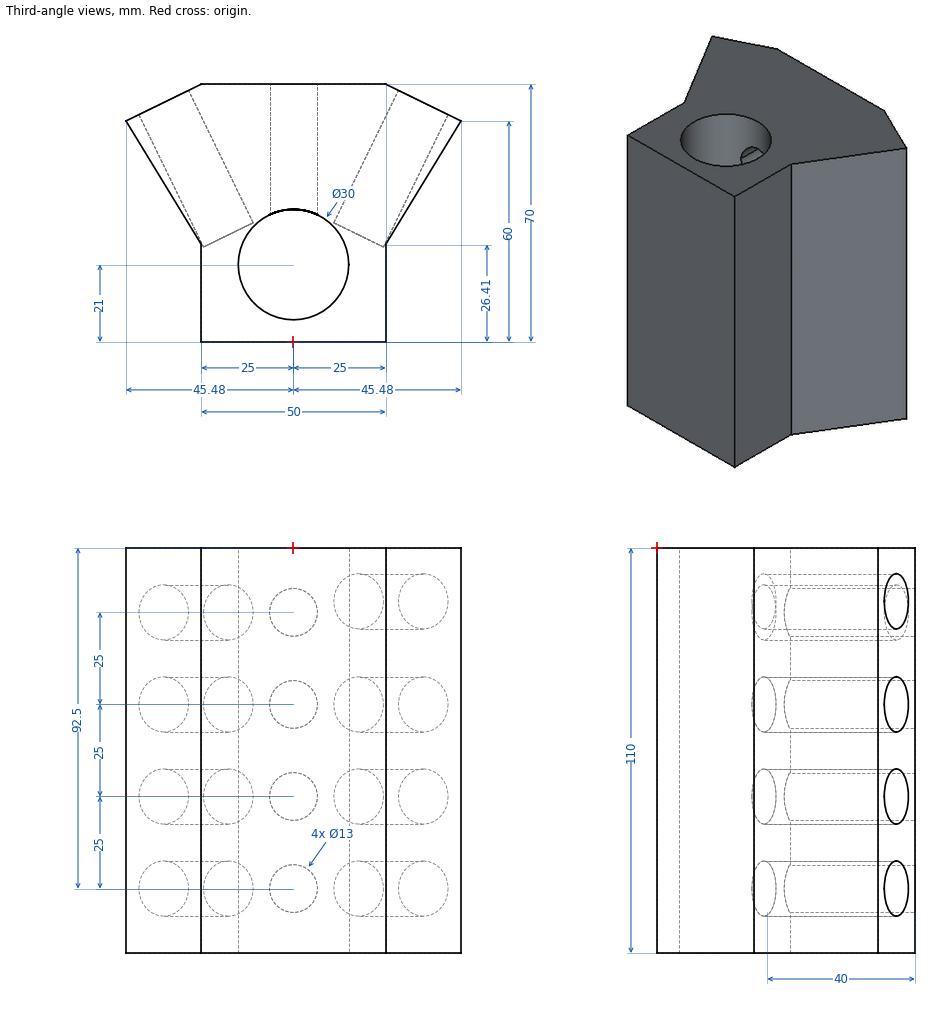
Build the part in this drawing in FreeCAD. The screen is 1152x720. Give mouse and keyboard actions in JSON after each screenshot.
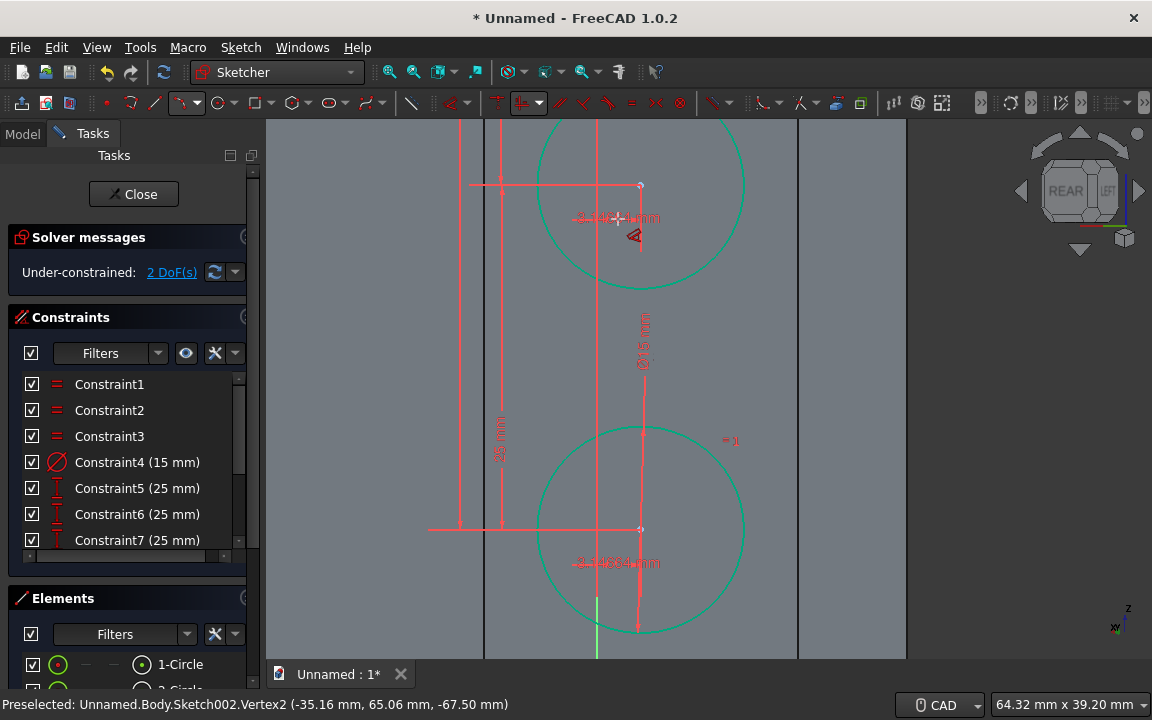
{"action": "scroll", "coordinate": [640, 535], "scroll_direction": "down", "scroll_amount": 7}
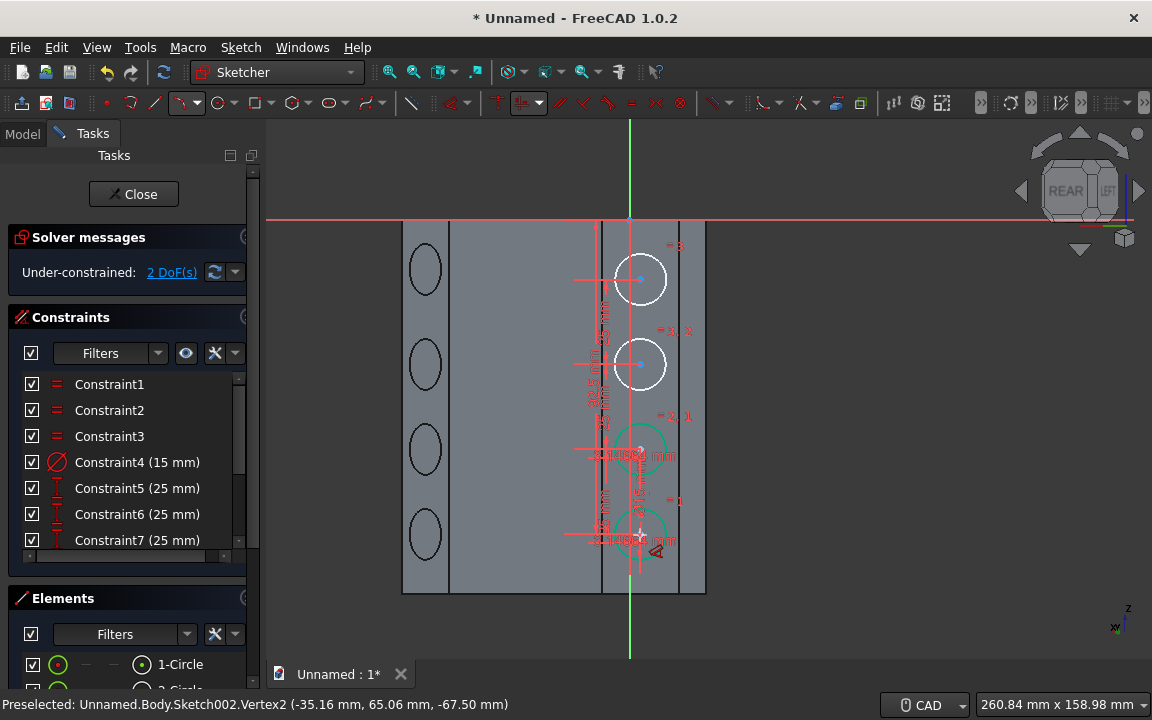
{"action": "scroll", "coordinate": [640, 364], "scroll_direction": "up", "scroll_amount": 7}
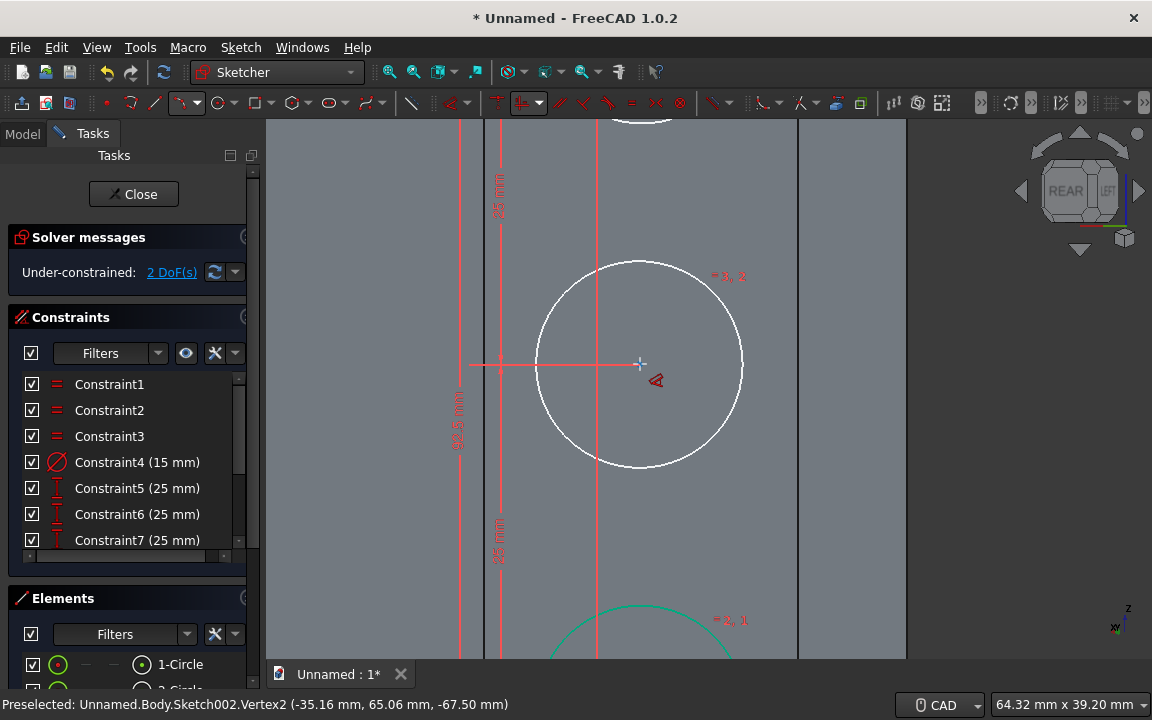
{"action": "left_click", "coordinate": [639, 365]}
{"action": "left_click", "coordinate": [618, 399]}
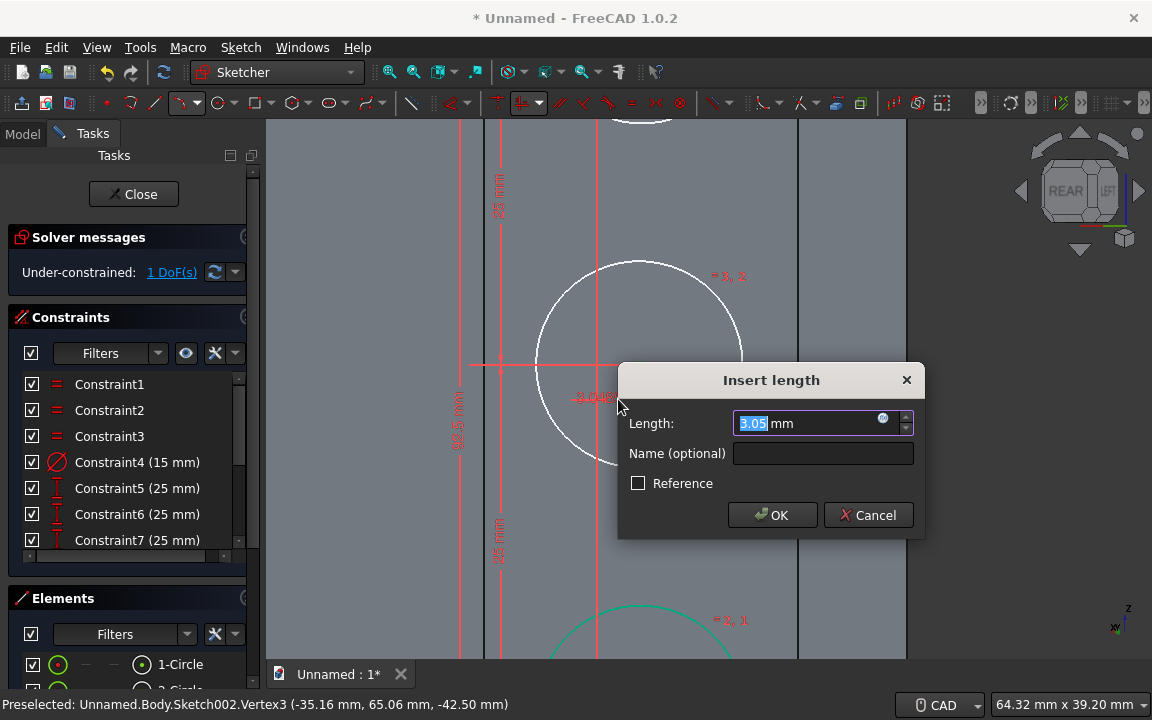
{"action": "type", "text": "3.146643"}
{"action": "key", "text": "Return"}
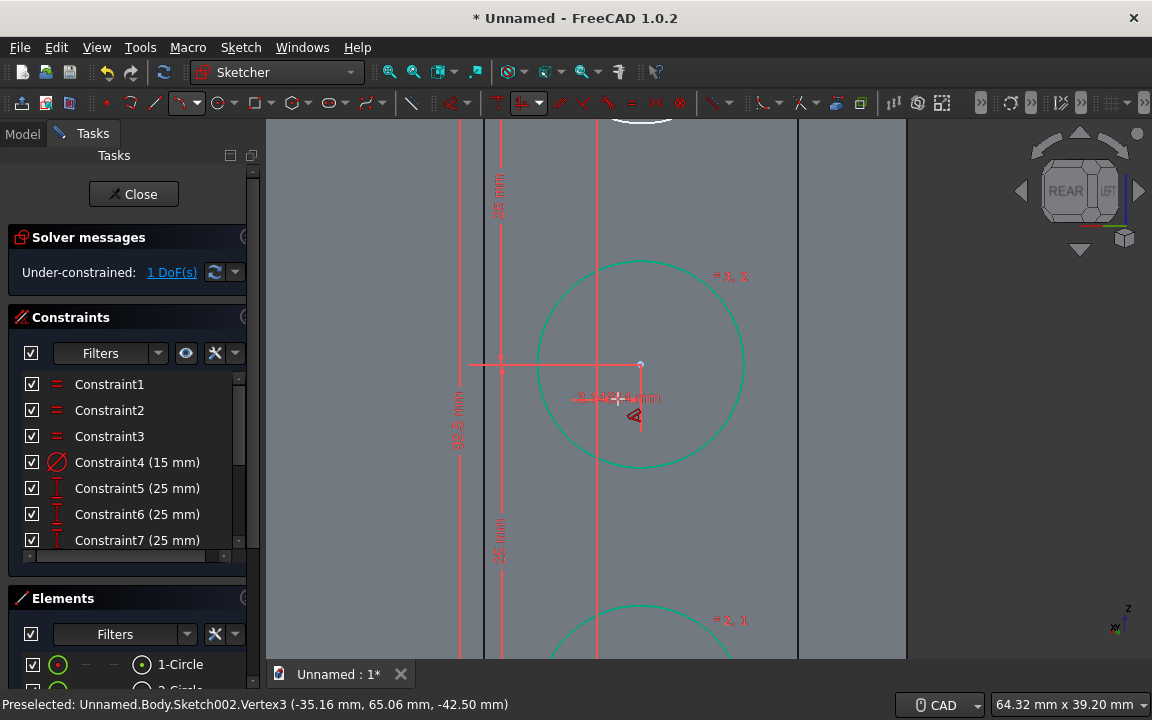
{"action": "scroll", "coordinate": [640, 363], "scroll_direction": "down", "scroll_amount": 7}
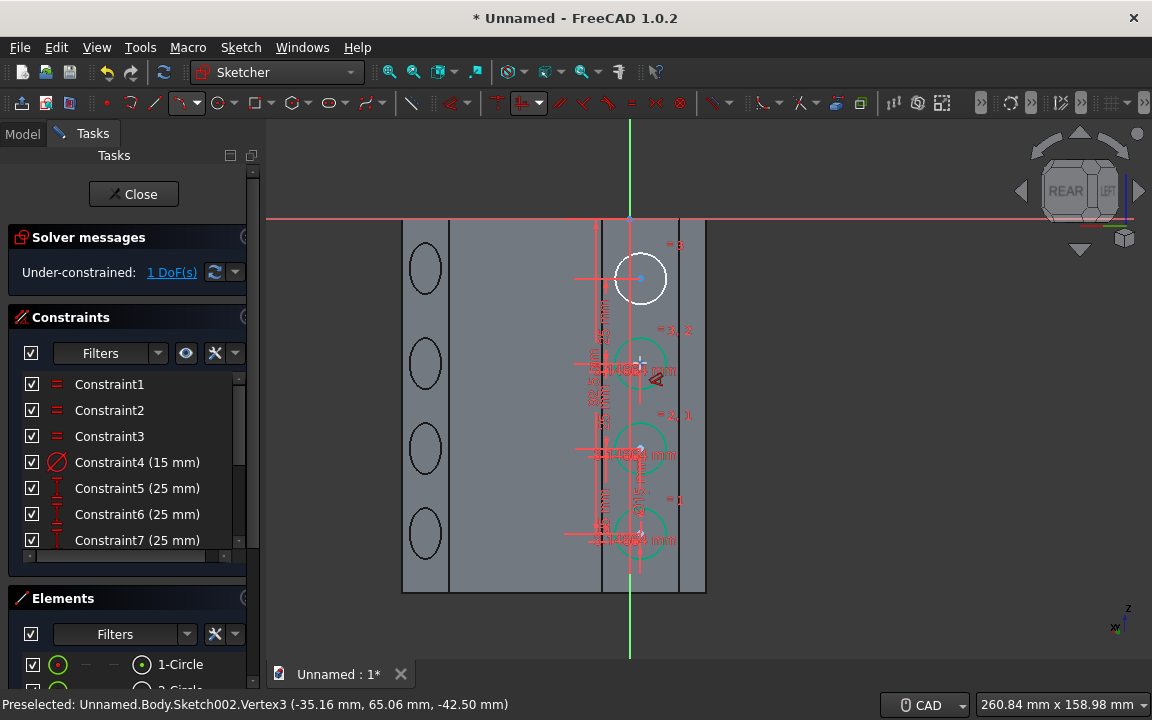
{"action": "scroll", "coordinate": [641, 279], "scroll_direction": "up", "scroll_amount": 7}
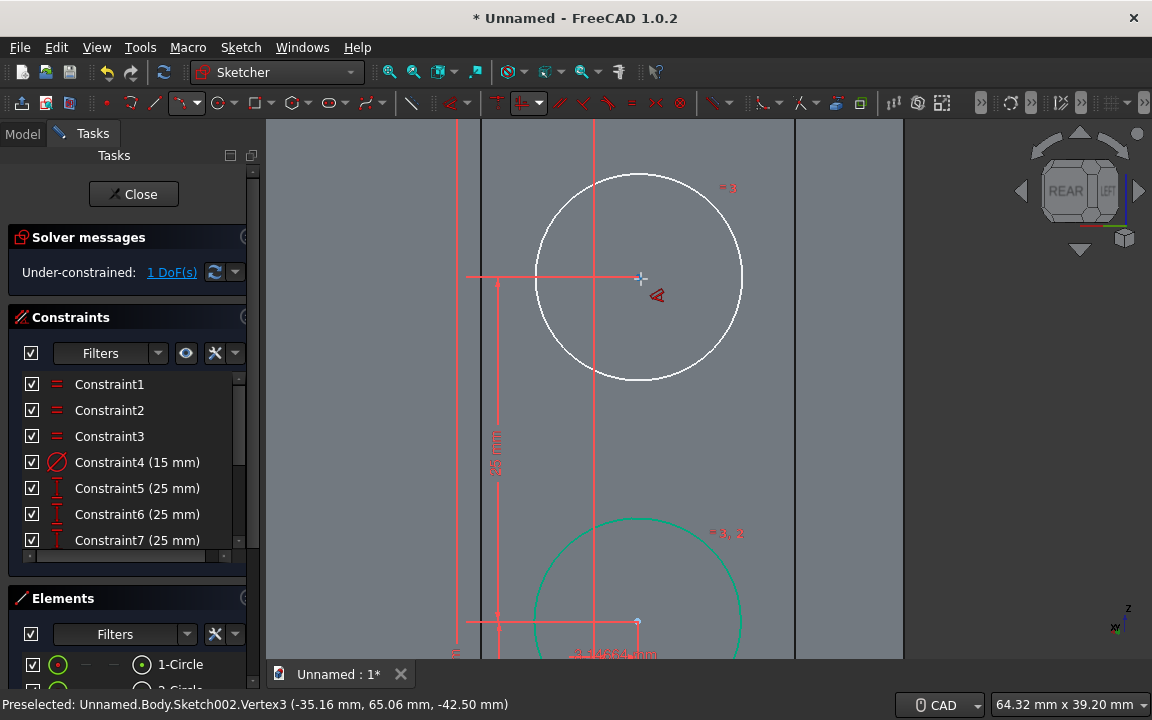
{"action": "left_click", "coordinate": [639, 277]}
{"action": "left_click", "coordinate": [617, 311]}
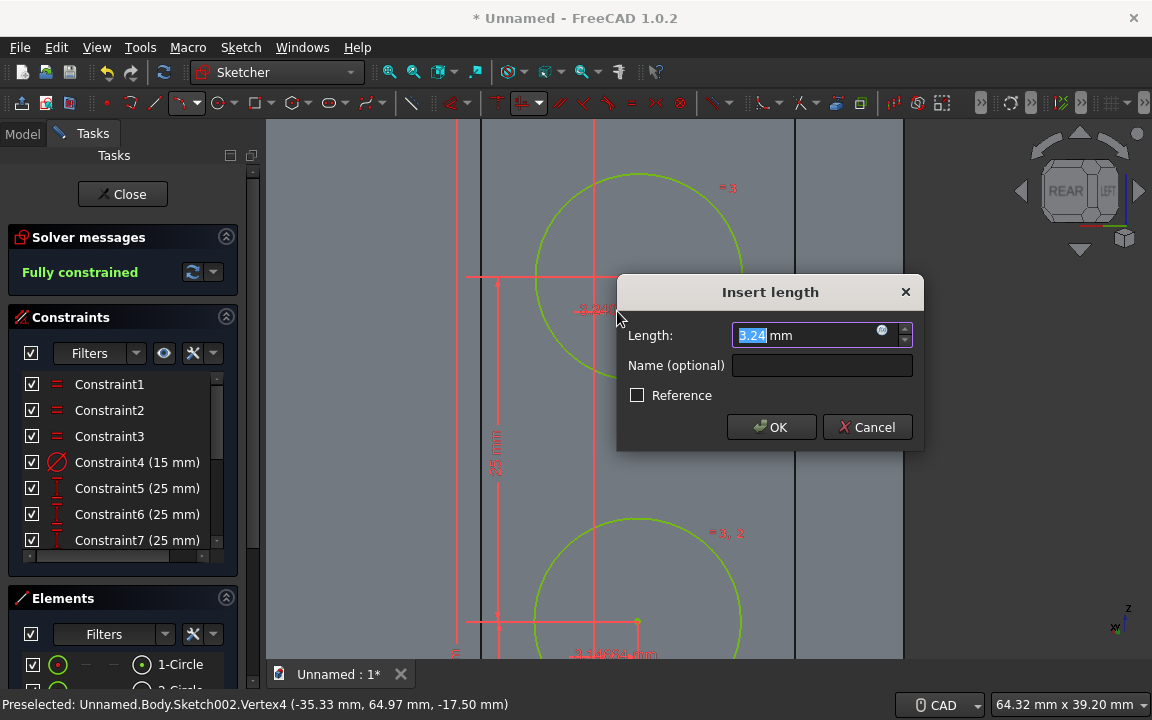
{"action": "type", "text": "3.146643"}
{"action": "key", "text": "Return"}
{"action": "key", "text": "Escape"}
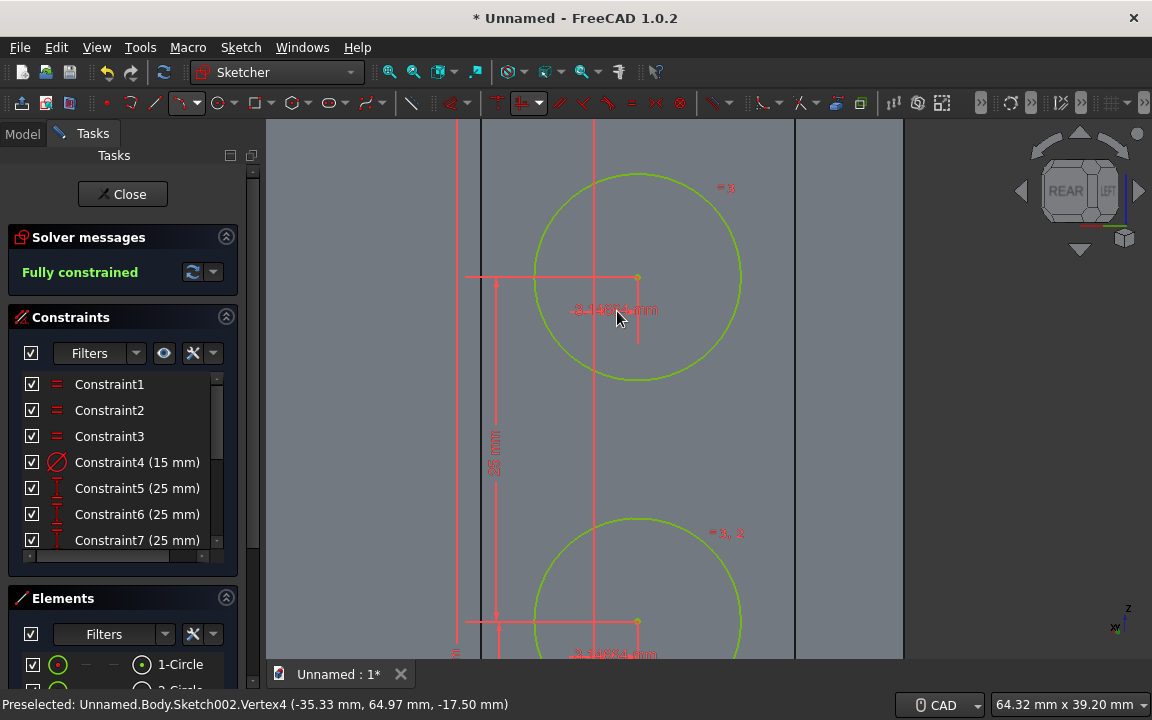
{"action": "left_click", "coordinate": [123, 194]}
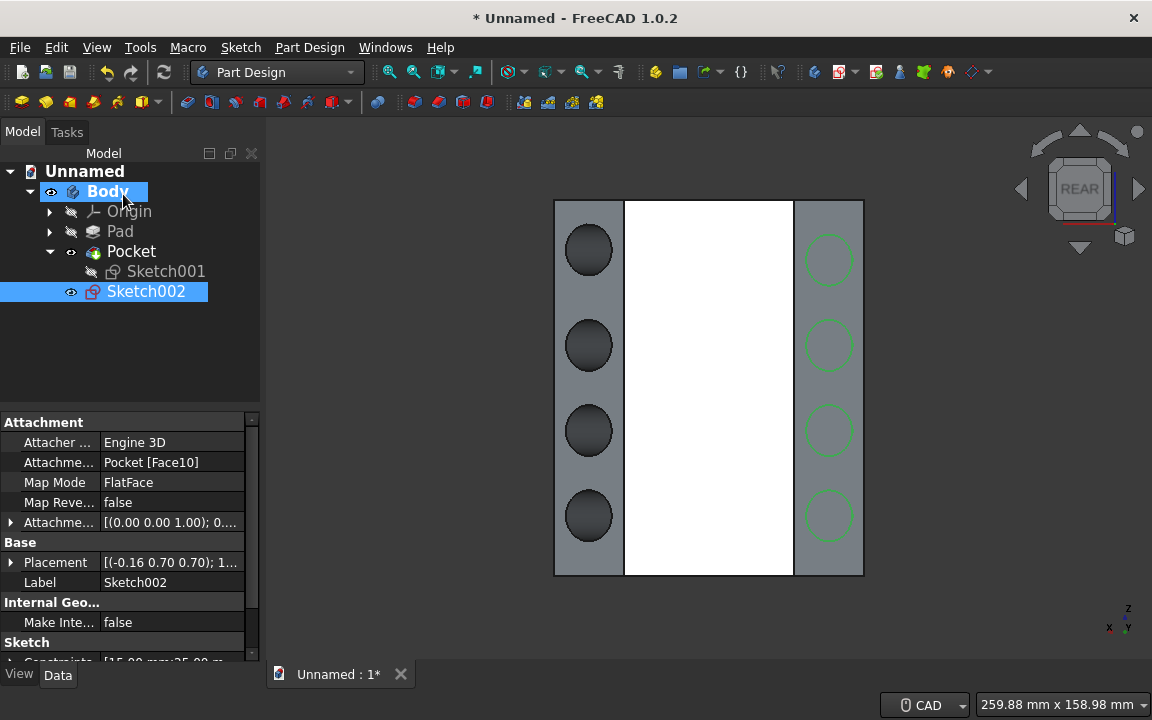
{"action": "left_click", "coordinate": [188, 102]}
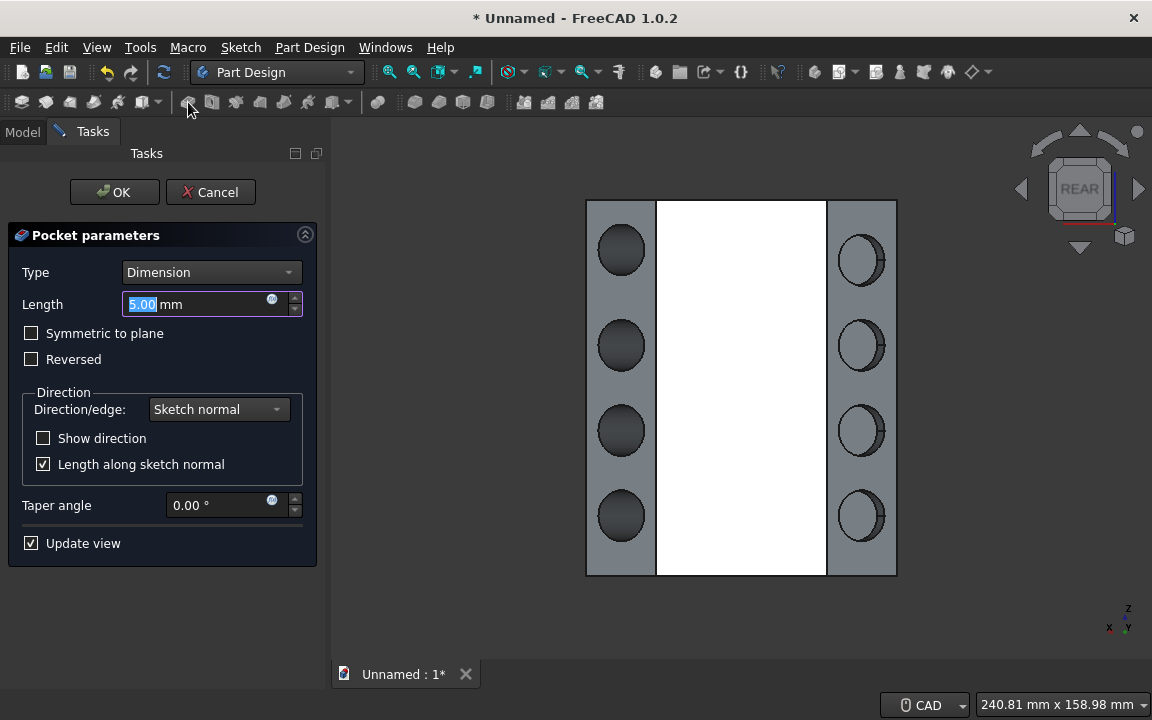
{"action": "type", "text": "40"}
{"action": "key", "text": "Tab"}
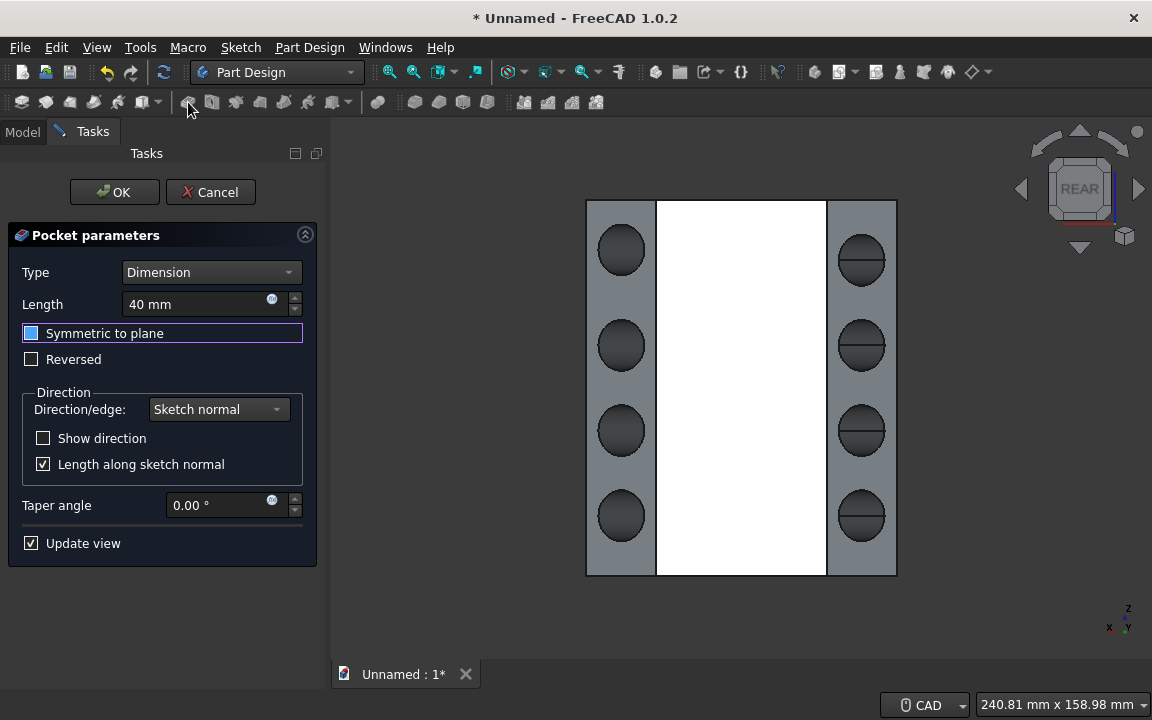
{"action": "left_click", "coordinate": [115, 192]}